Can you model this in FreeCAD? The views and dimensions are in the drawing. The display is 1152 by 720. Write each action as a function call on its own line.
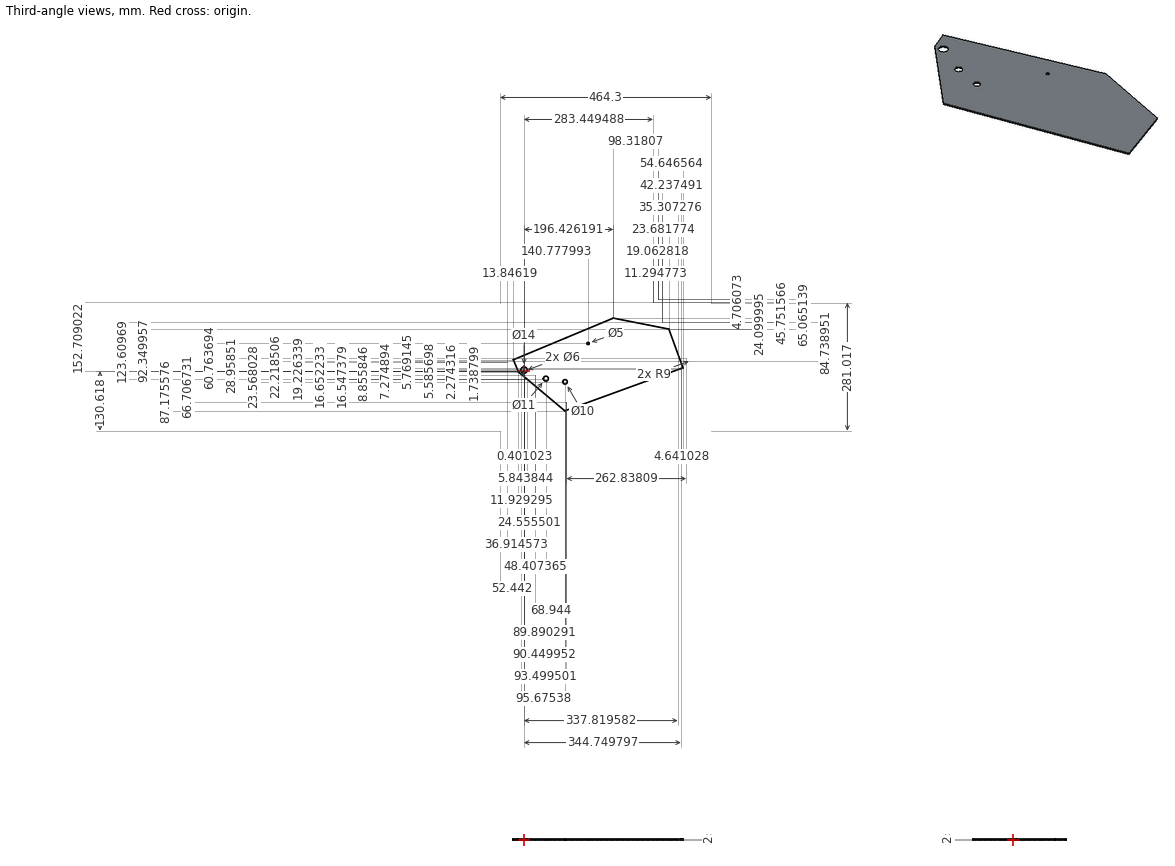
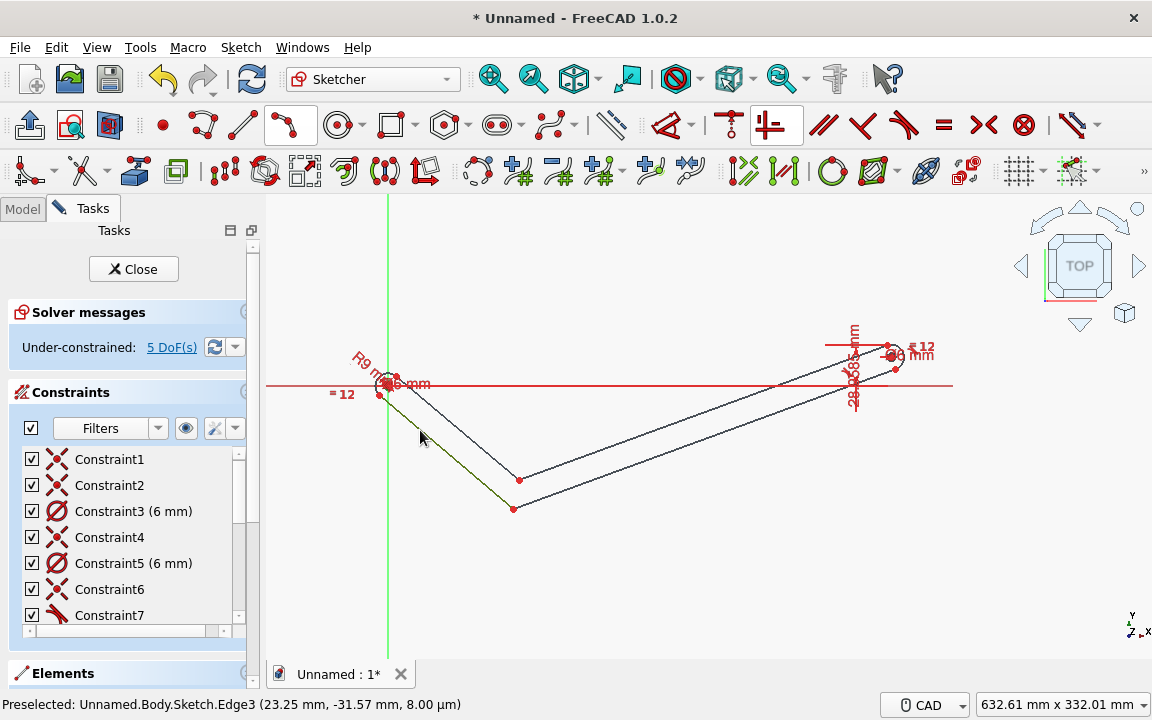
key(l)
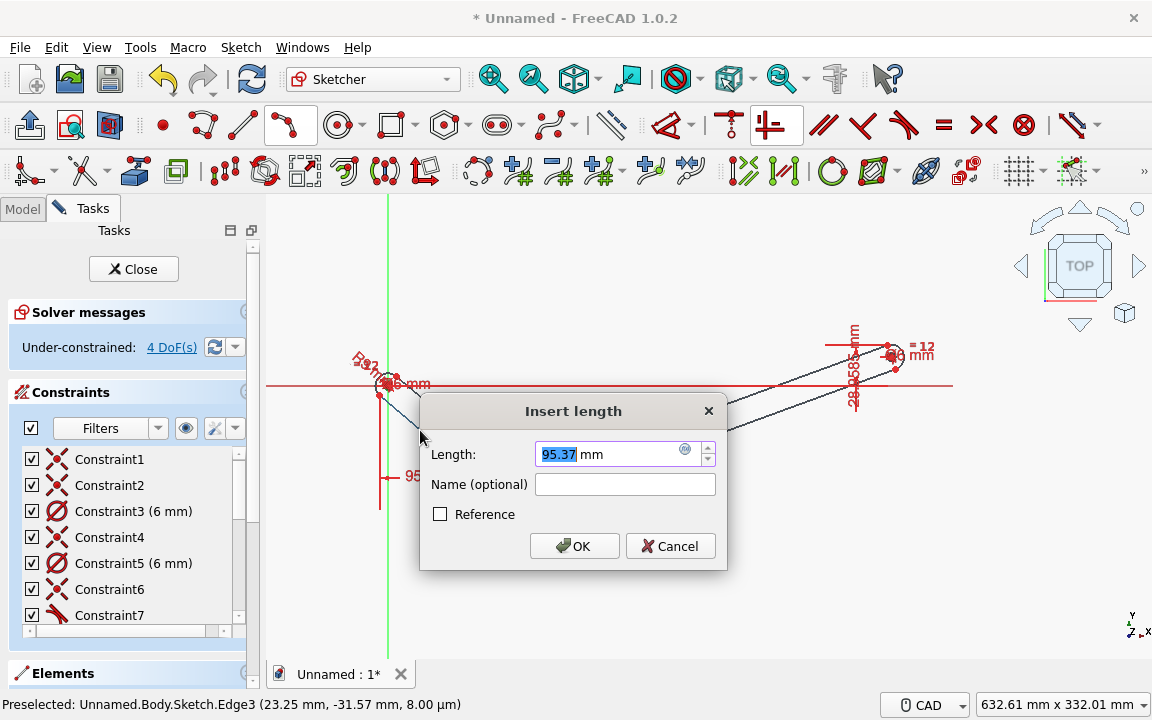
text(95.67538)
key(Return)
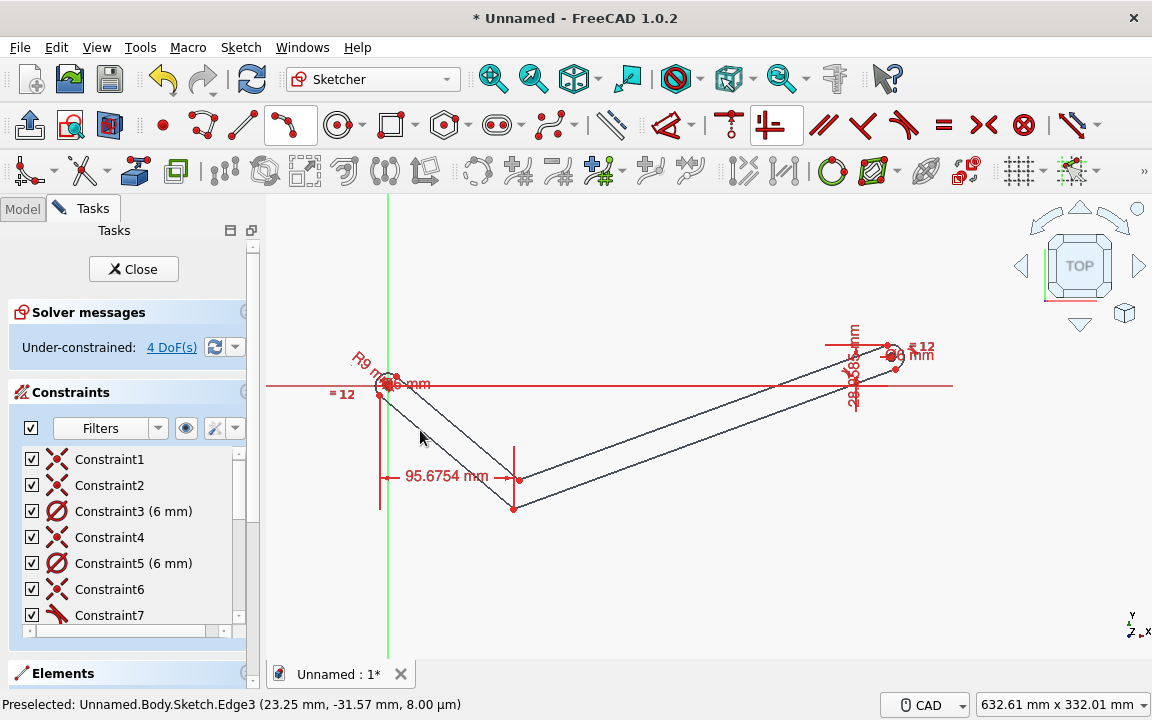
click(519, 480)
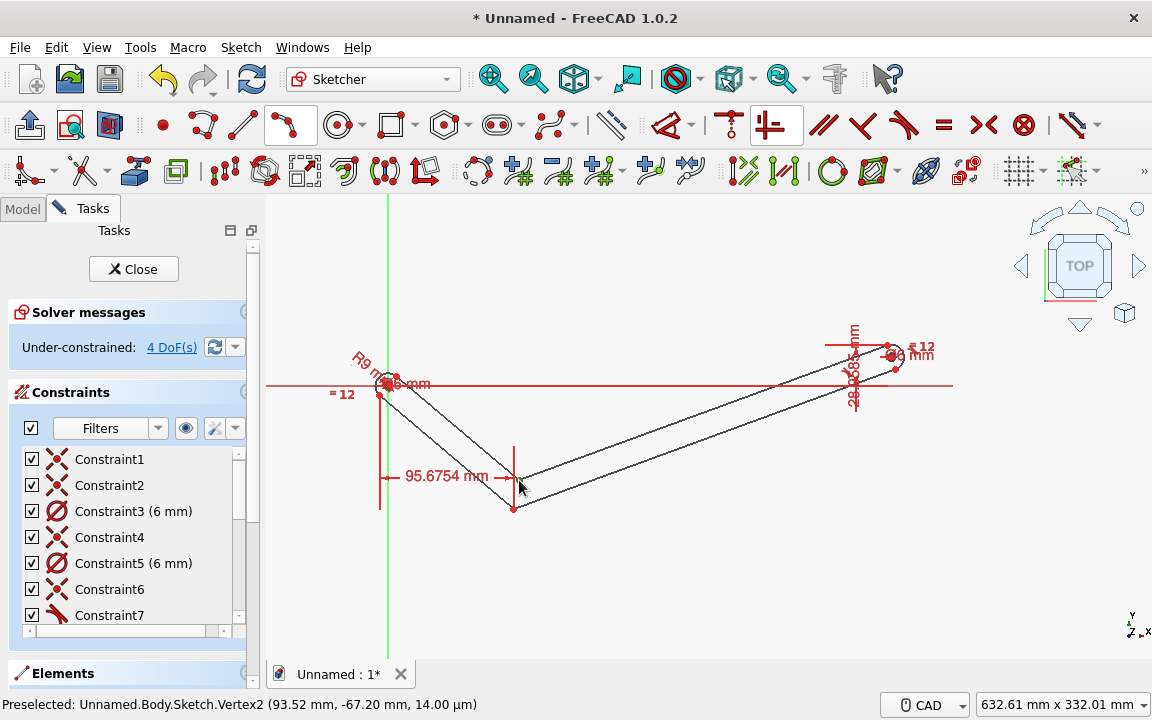
key(l)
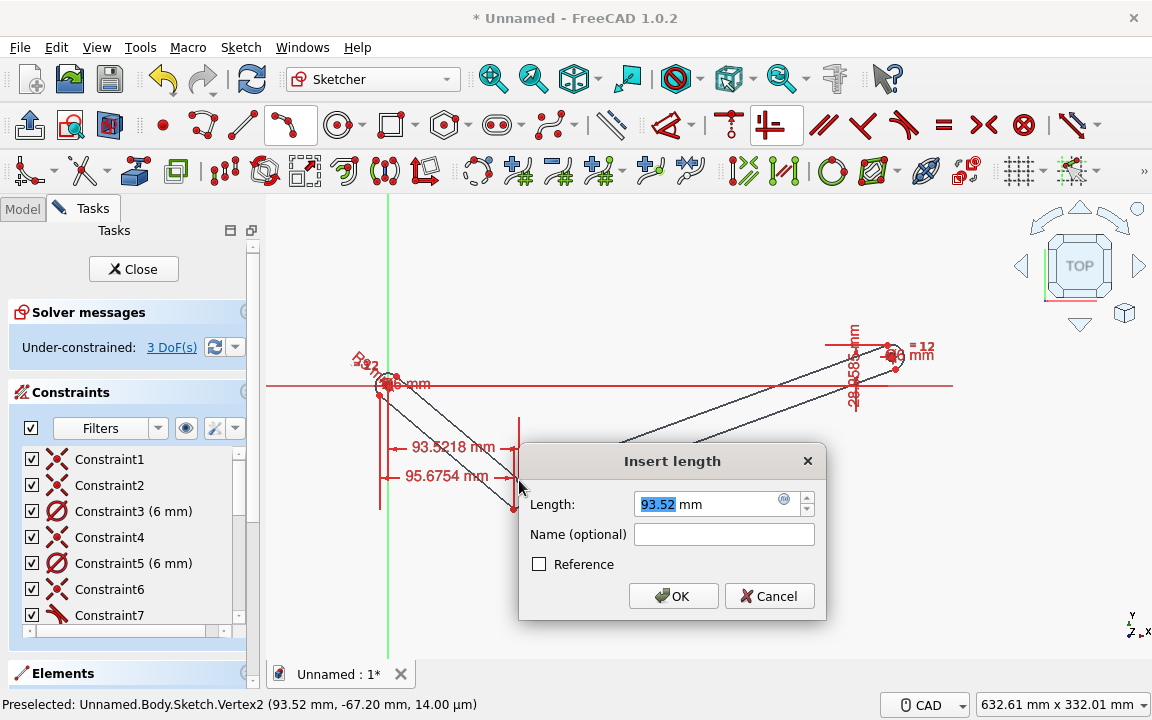
text(93.499501)
key(Return)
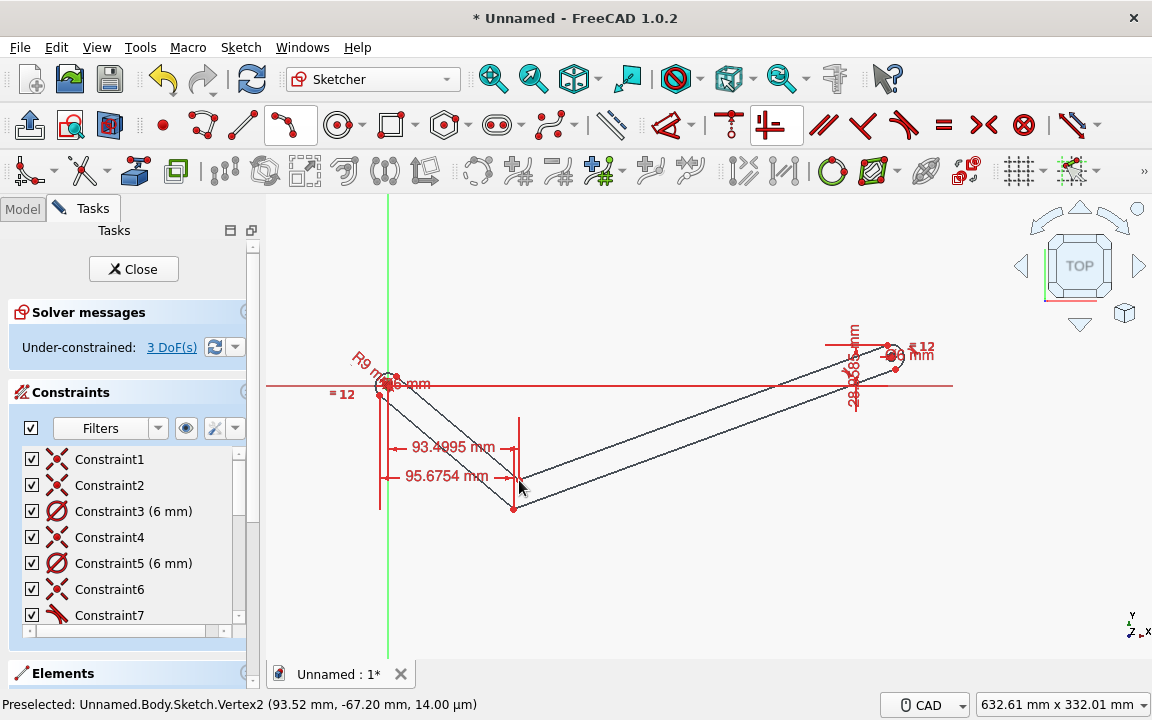
click(519, 480)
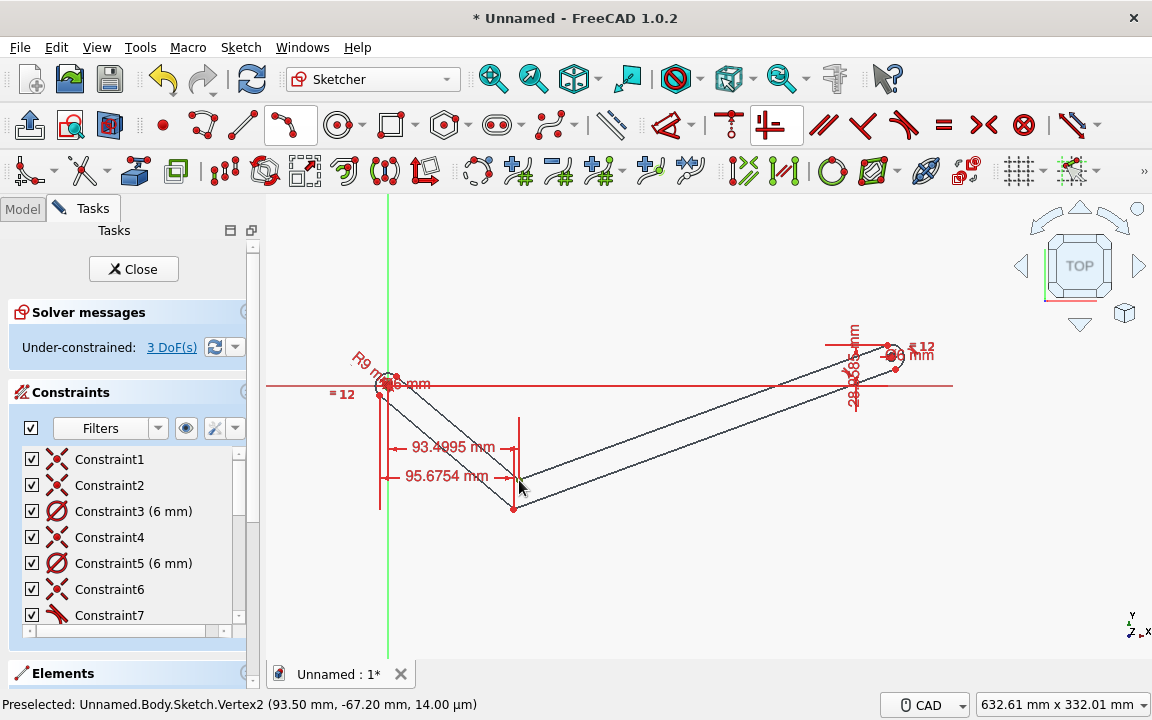
key(i)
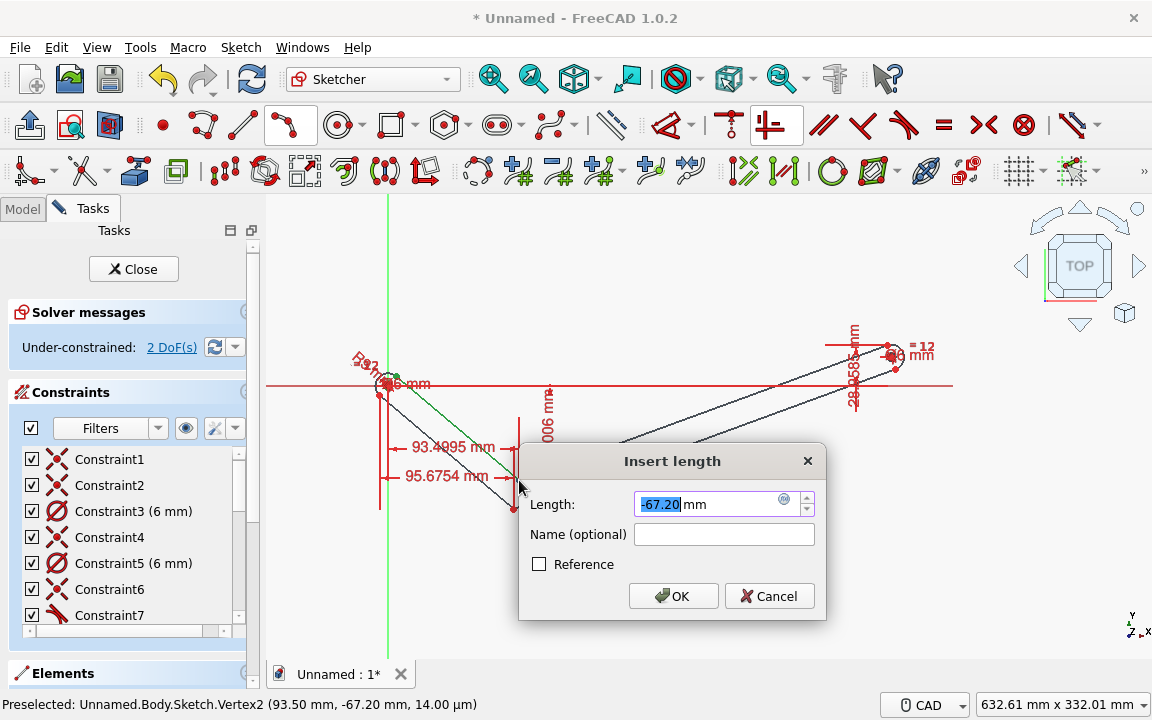
text(-66.706731)
key(Return)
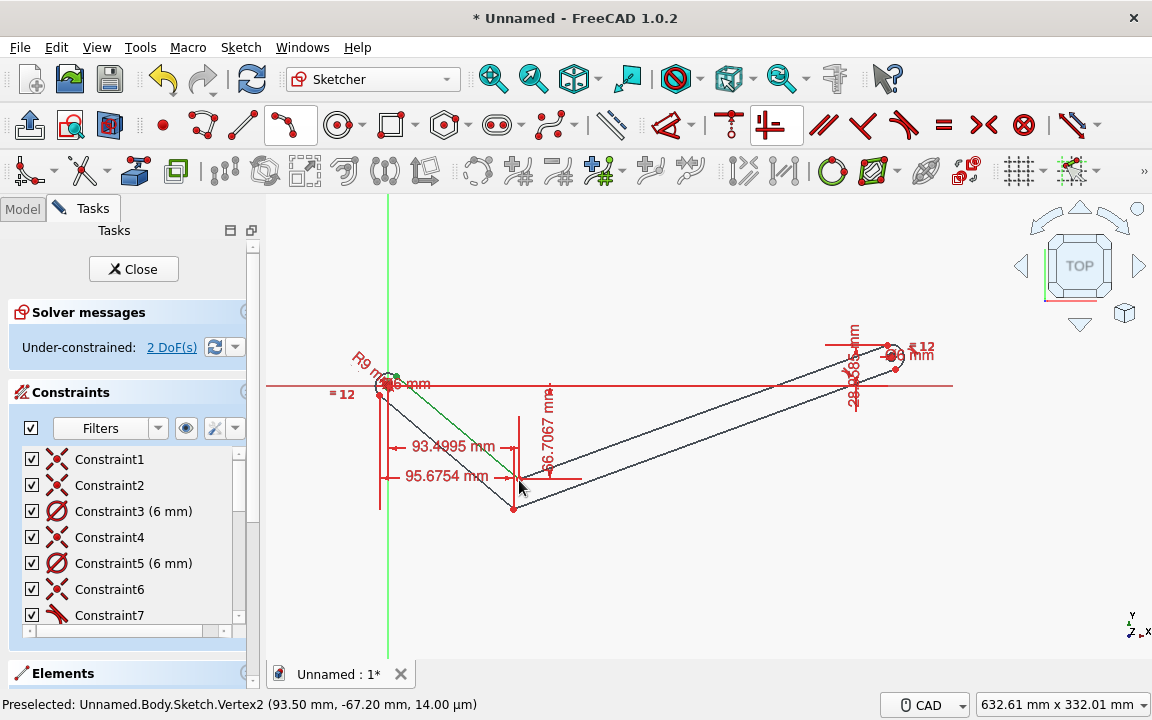
click(514, 509)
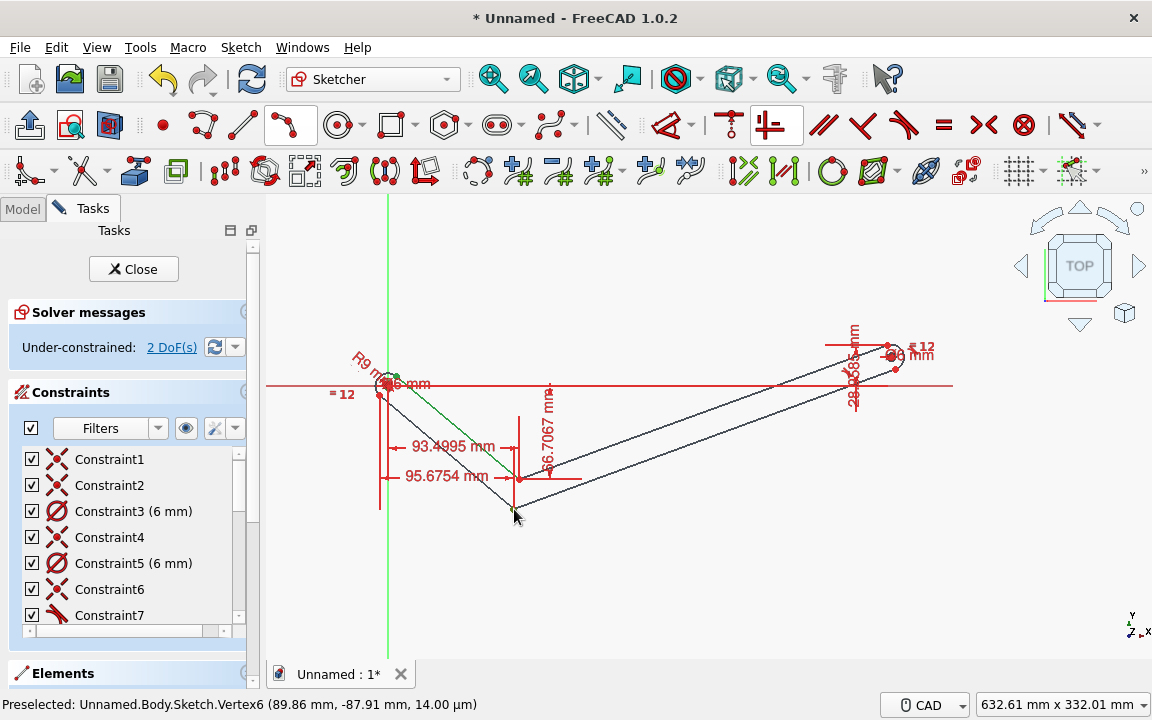
key(i)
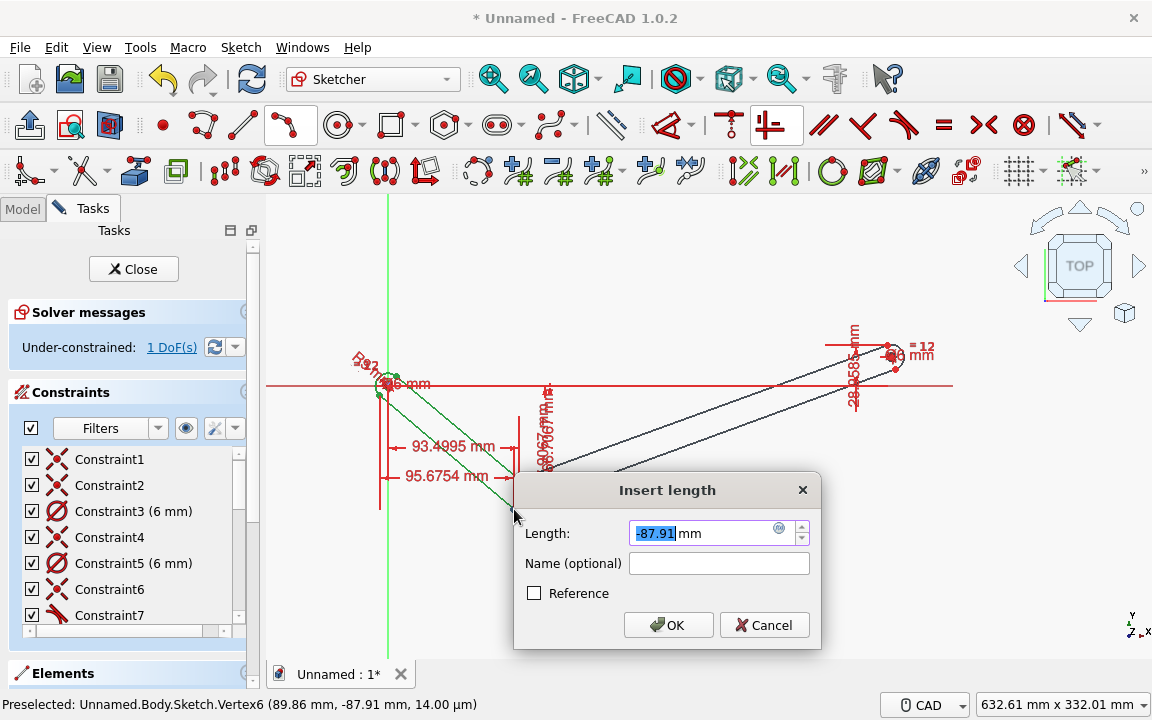
text(-87.175576)
key(Return)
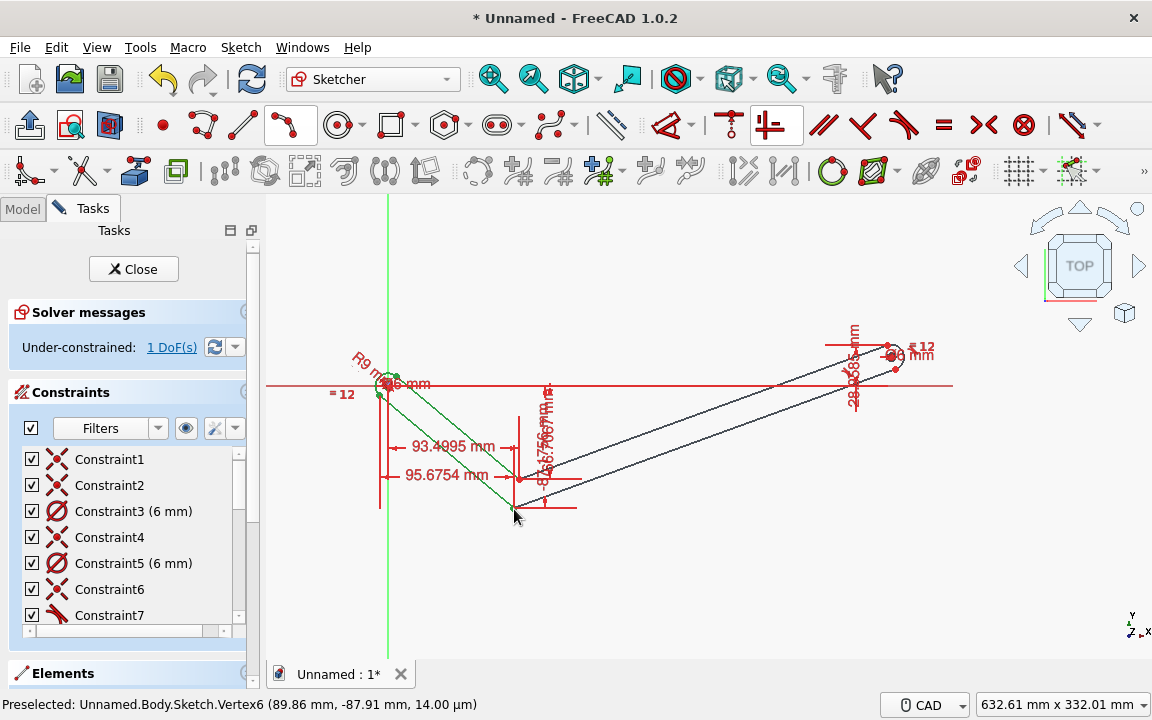
click(777, 386)